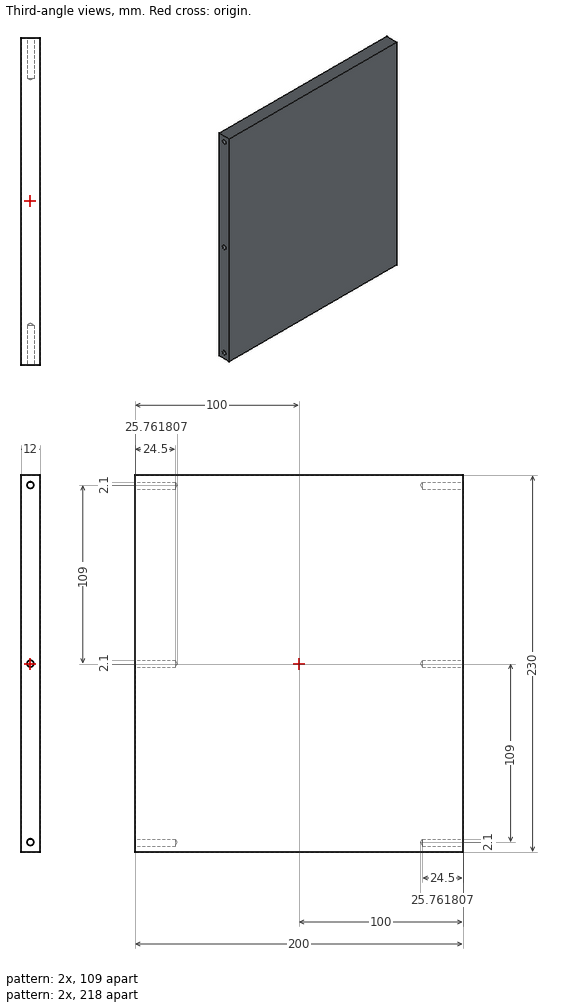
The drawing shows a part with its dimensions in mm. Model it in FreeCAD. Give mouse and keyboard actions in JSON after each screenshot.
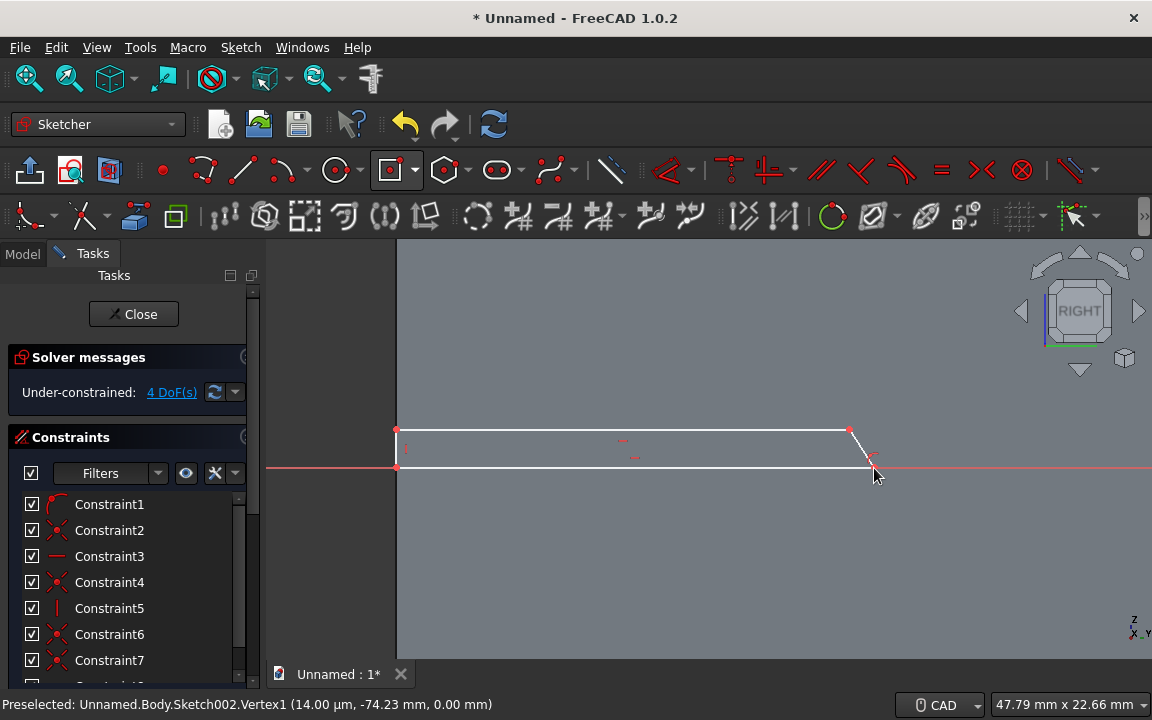
{"action": "left_click", "coordinate": [666, 170]}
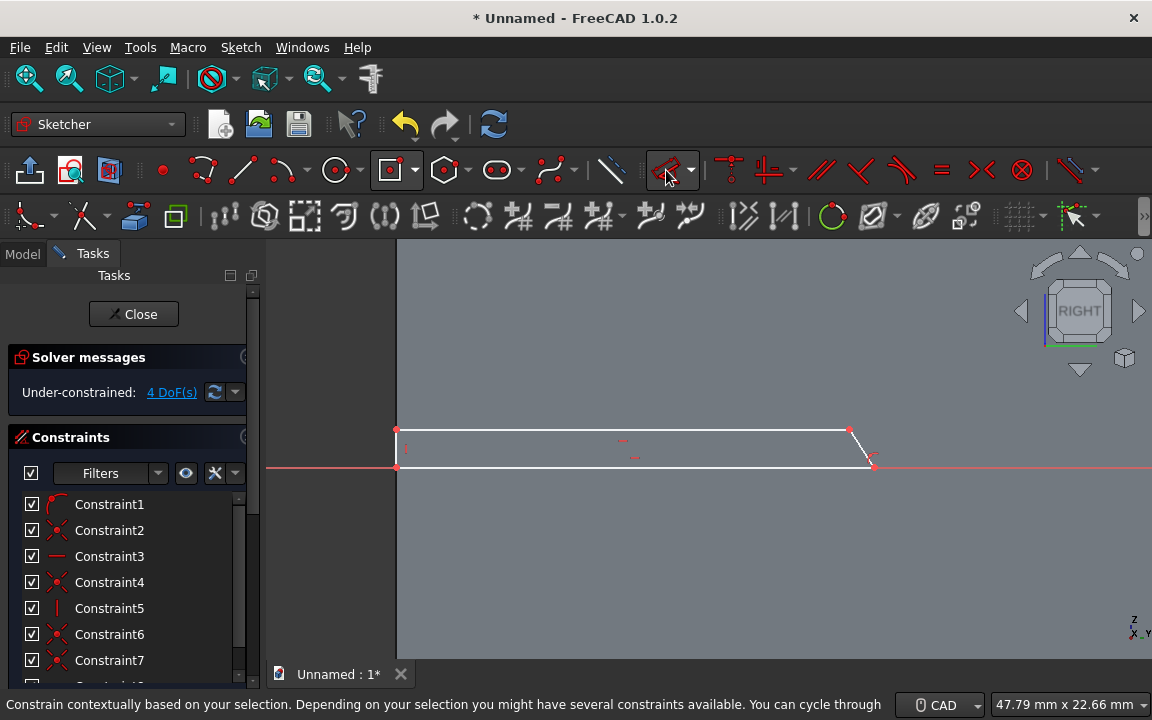
{"action": "left_click", "coordinate": [396, 441]}
{"action": "left_click", "coordinate": [362, 449]}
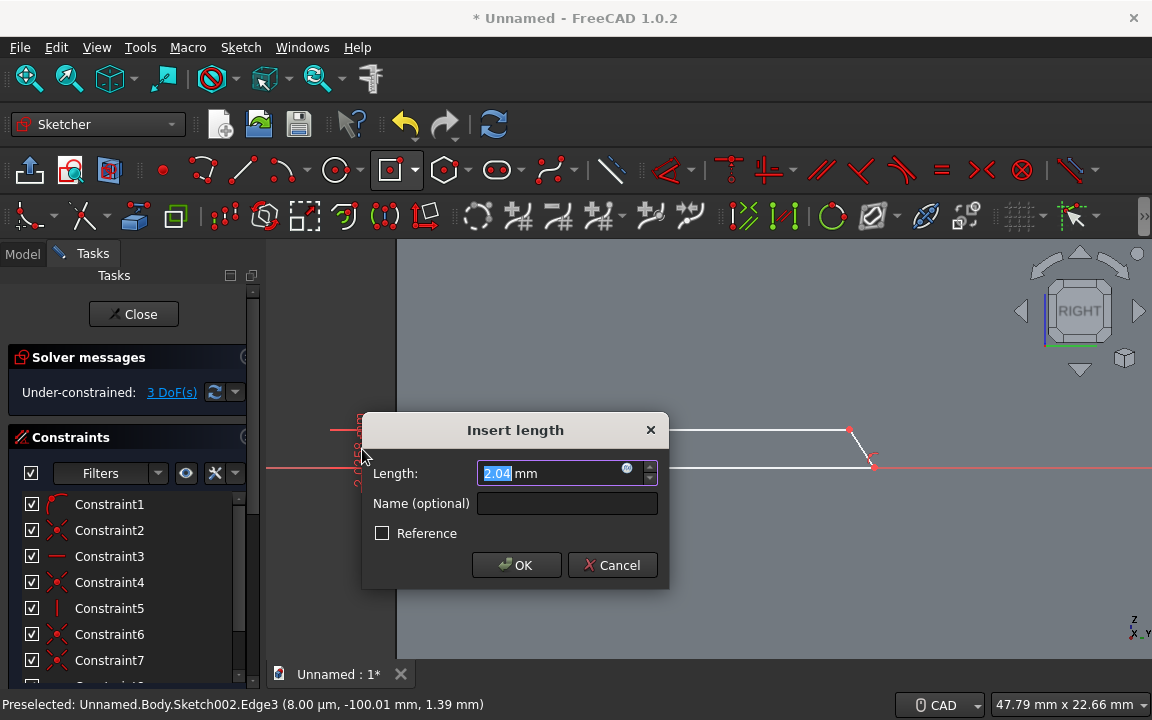
{"action": "type", "text": "2.1"}
{"action": "key", "text": "Return"}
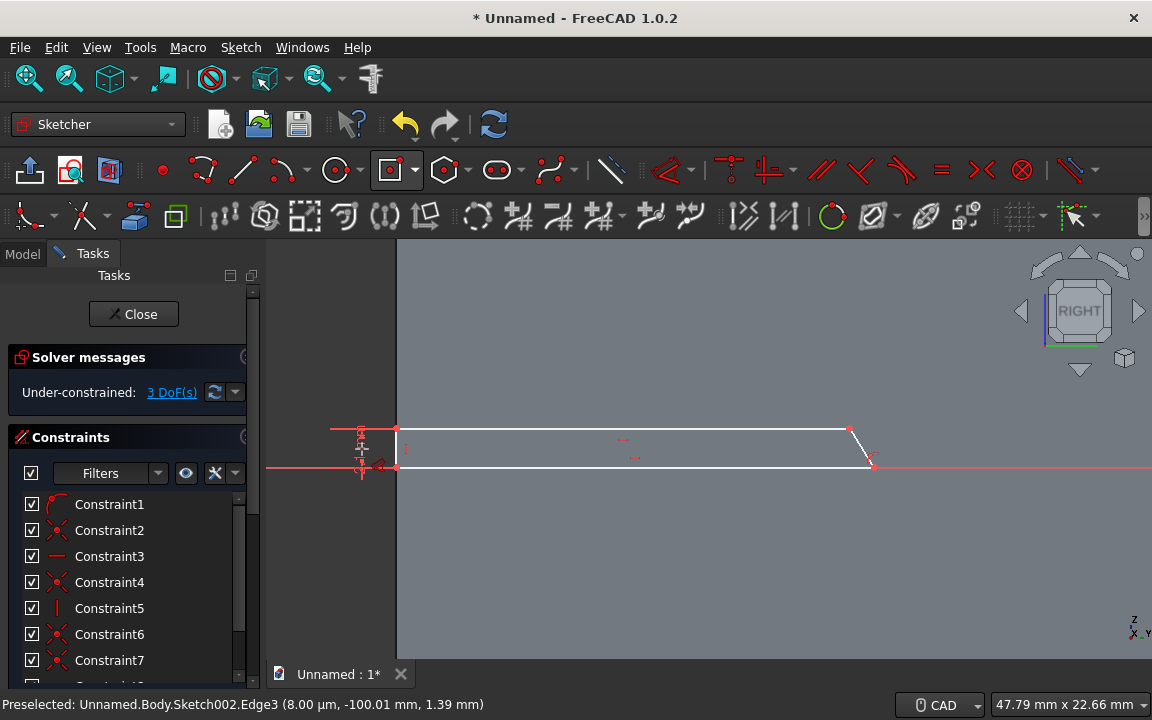
{"action": "left_click", "coordinate": [714, 429]}
{"action": "left_click", "coordinate": [623, 395]}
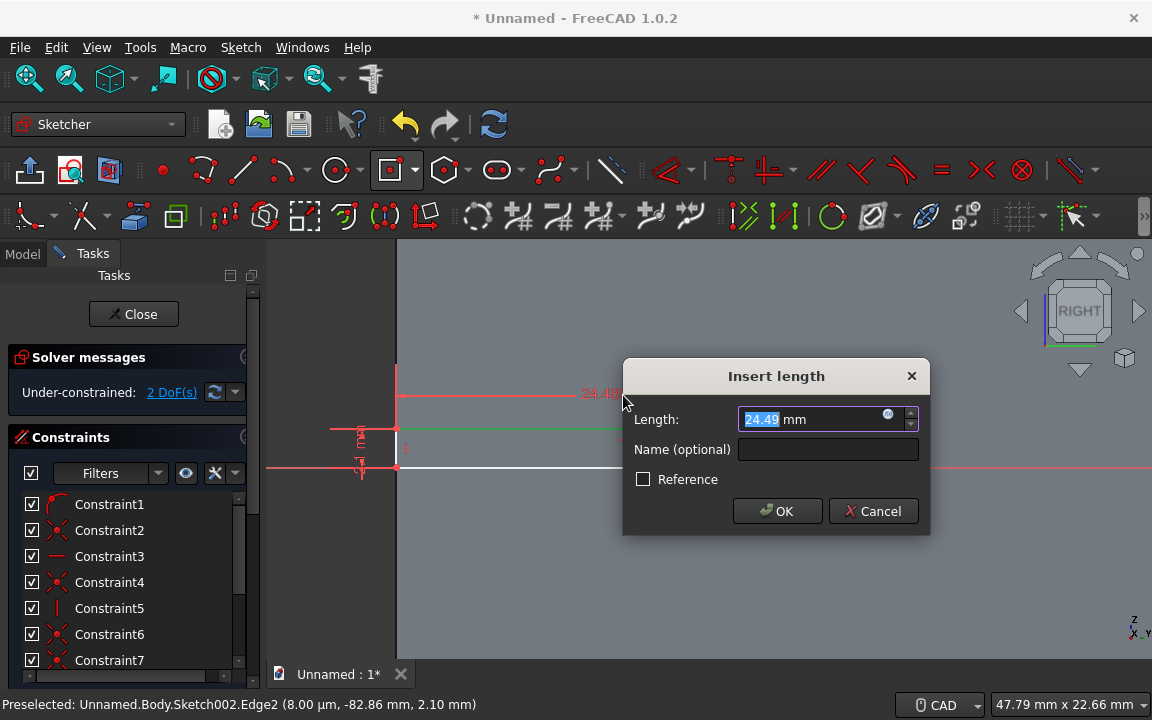
{"action": "type", "text": "24.5"}
{"action": "key", "text": "Return"}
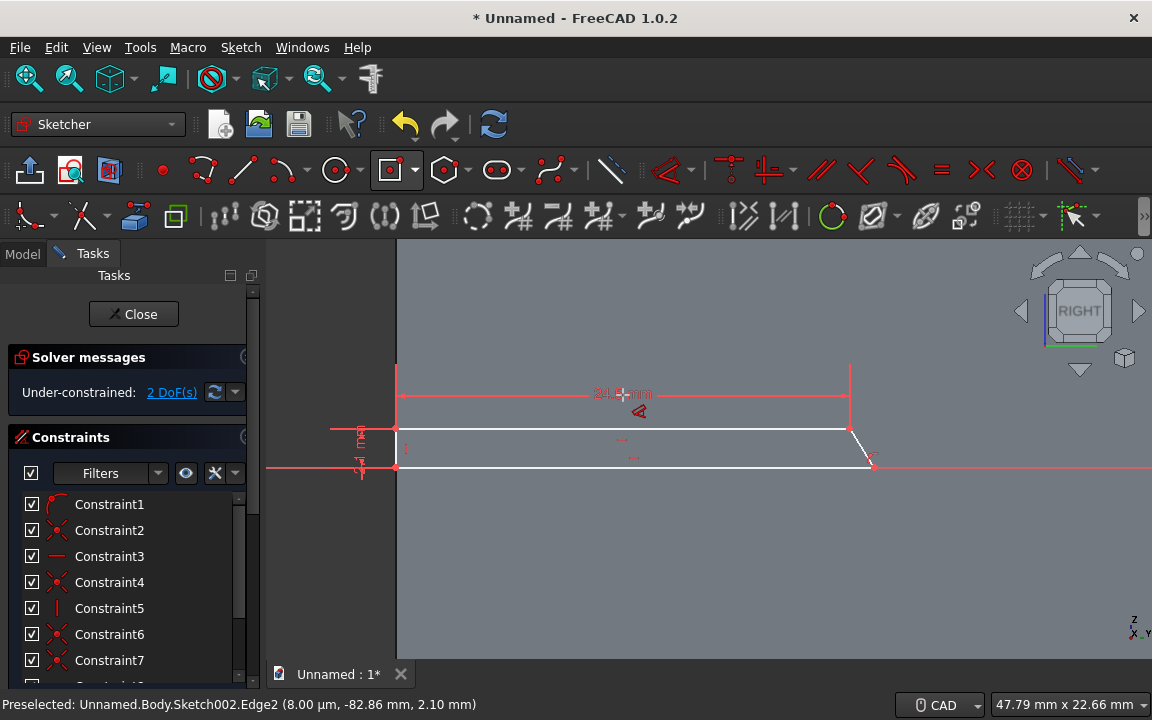
{"action": "left_click", "coordinate": [396, 429]}
{"action": "left_click", "coordinate": [691, 502]}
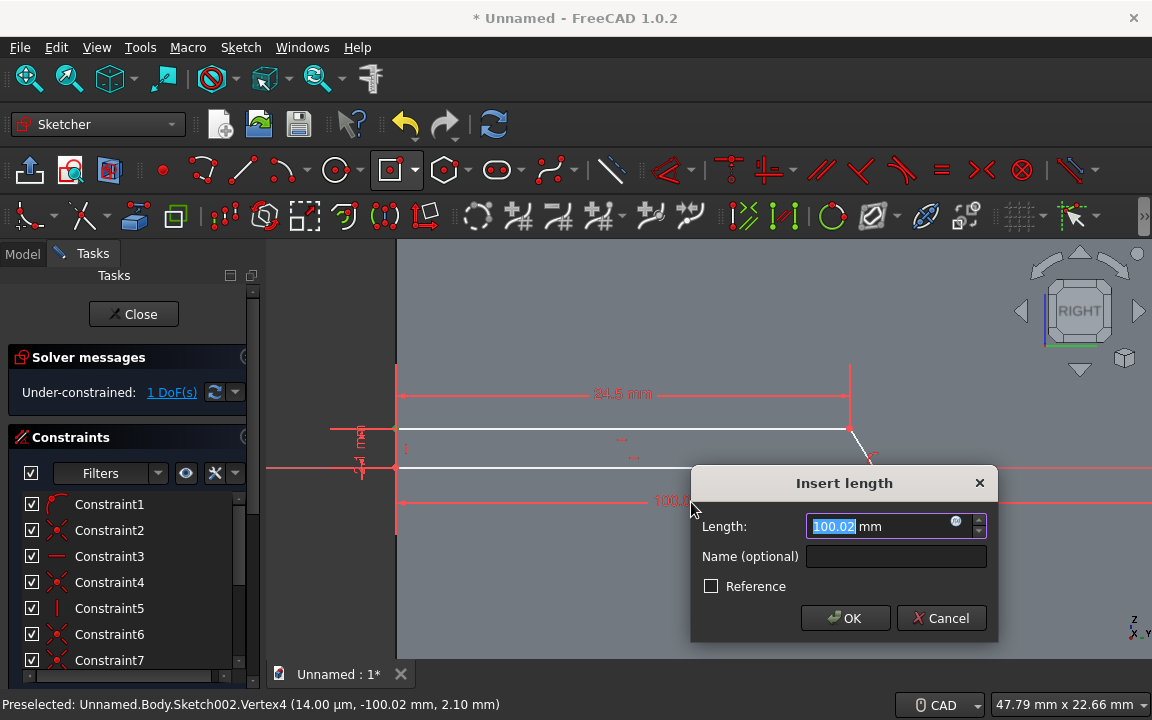
{"action": "type", "text": "100"}
{"action": "key", "text": "Return"}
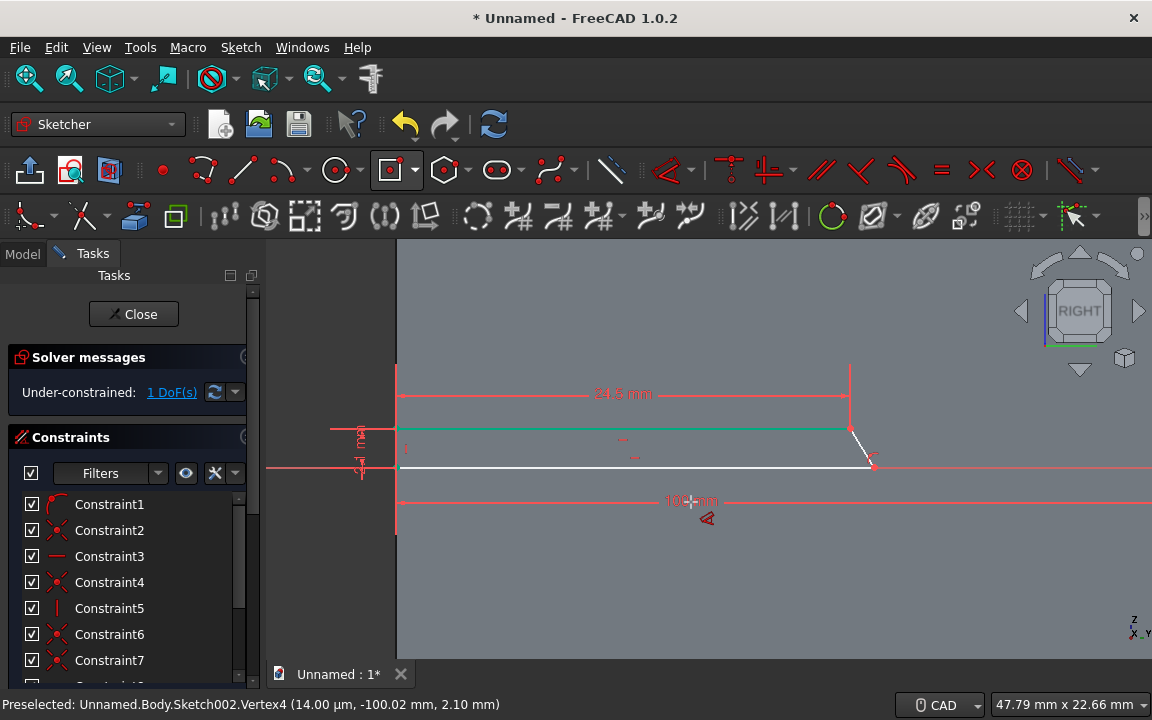
{"action": "left_click", "coordinate": [540, 468]}
{"action": "left_click", "coordinate": [525, 502]}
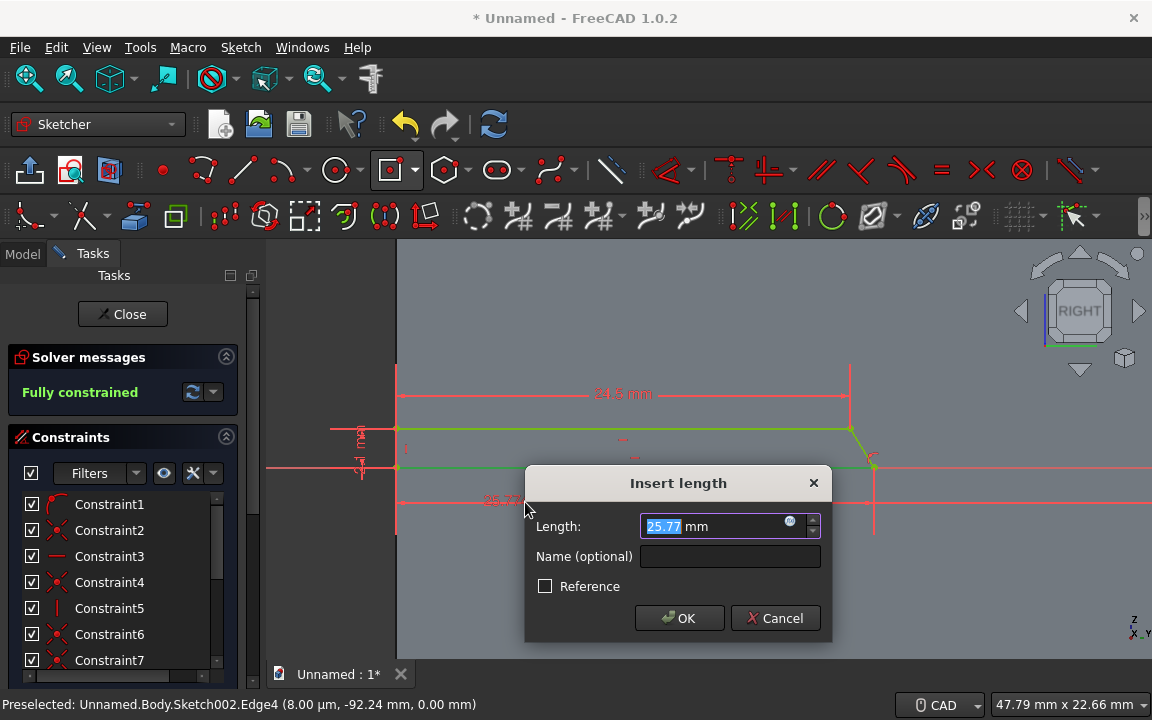
{"action": "type", "text": "25.761807"}
{"action": "key", "text": "Return"}
{"action": "key", "text": "Escape"}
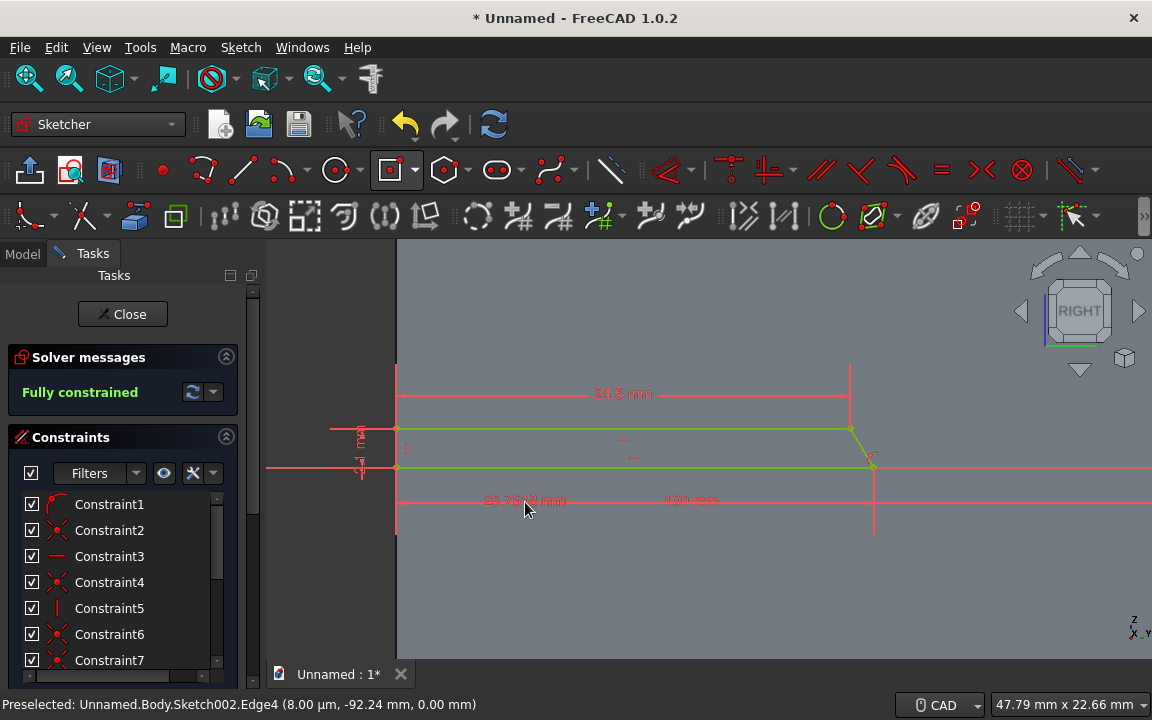
{"action": "left_click", "coordinate": [123, 314]}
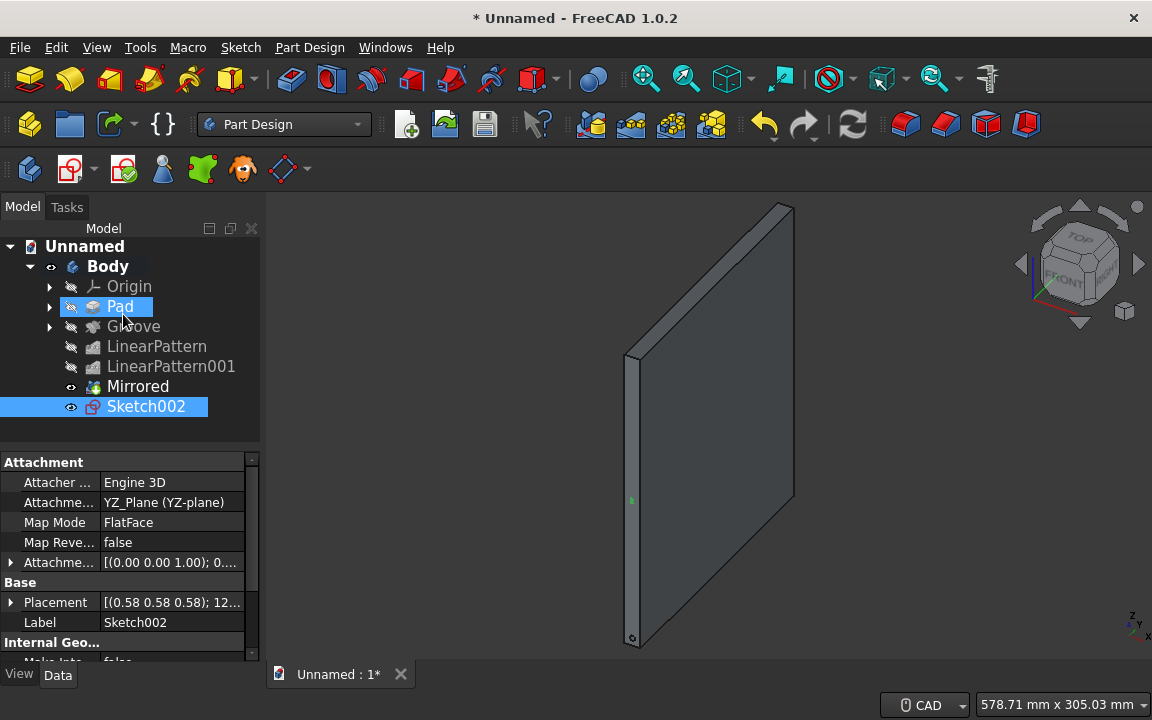
{"action": "left_click", "coordinate": [372, 80]}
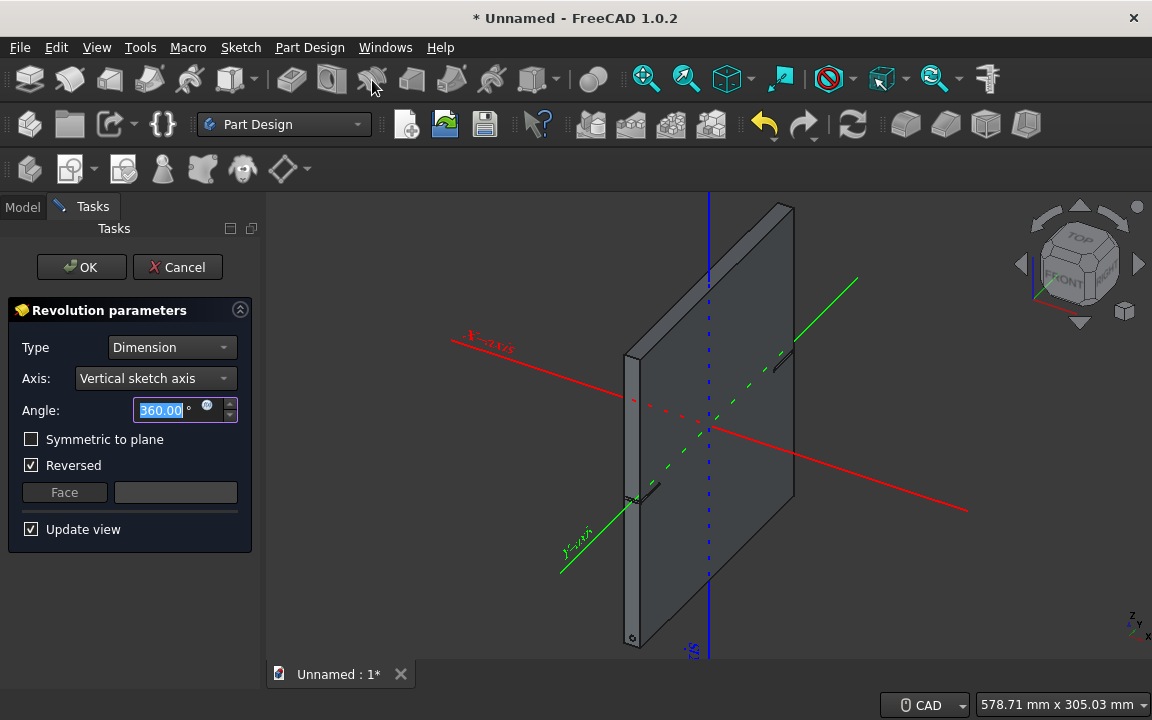
{"action": "left_click", "coordinate": [156, 378]}